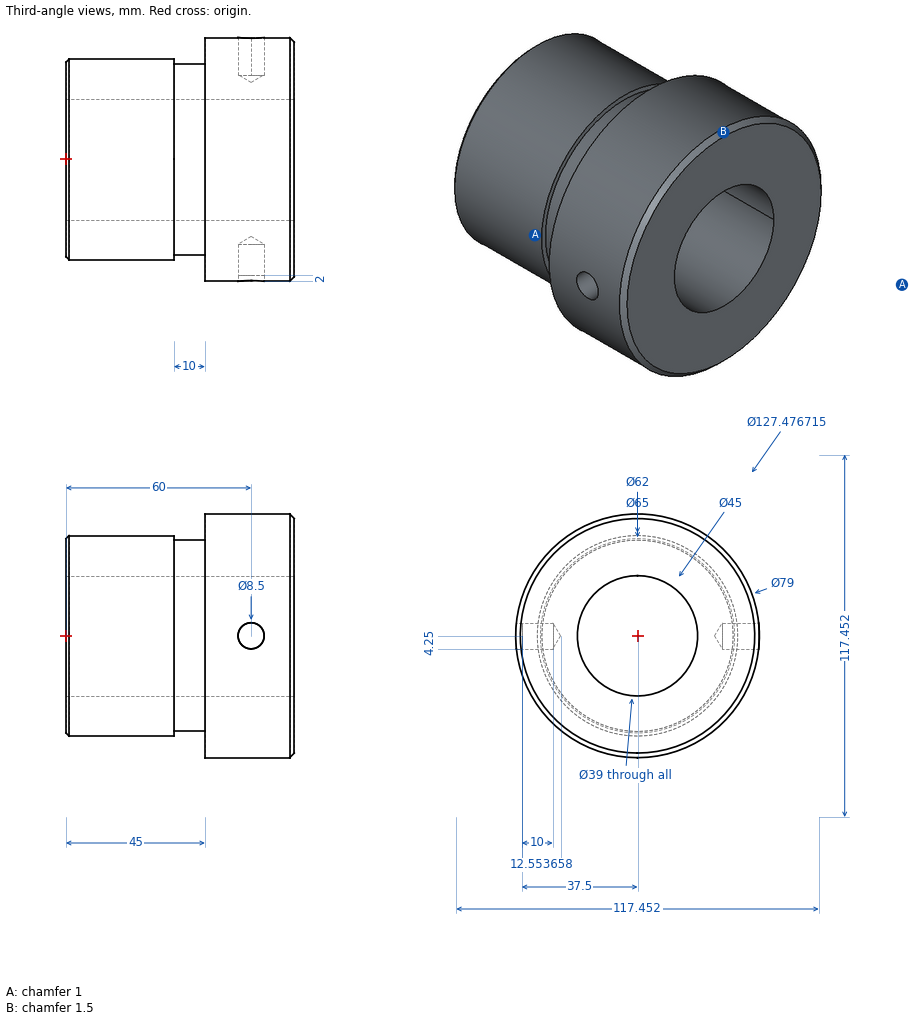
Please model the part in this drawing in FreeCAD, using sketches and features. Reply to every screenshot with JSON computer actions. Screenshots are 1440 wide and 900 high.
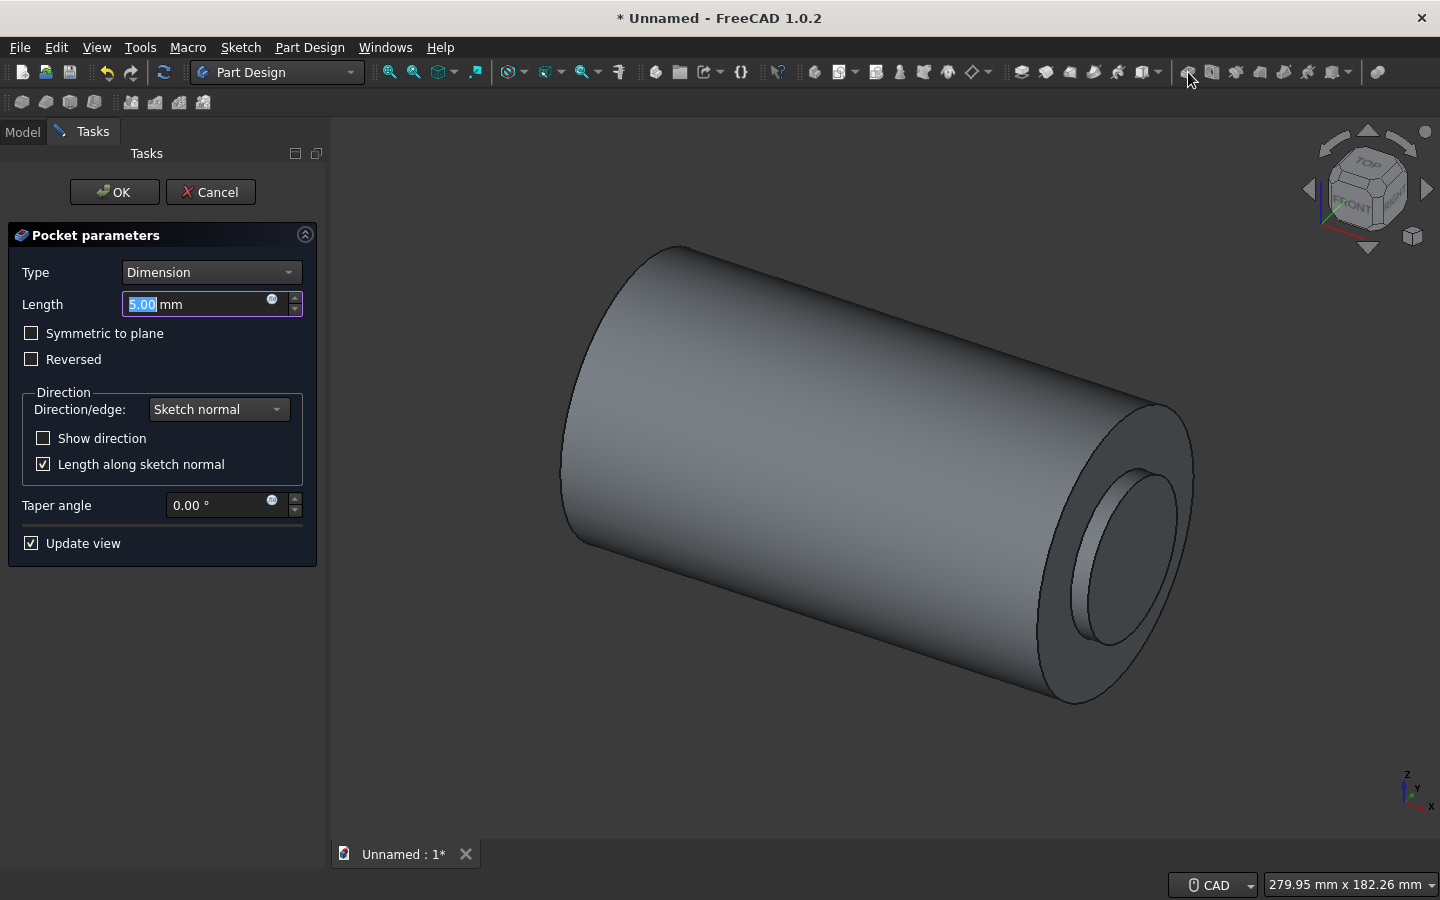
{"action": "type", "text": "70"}
{"action": "key", "text": "Tab"}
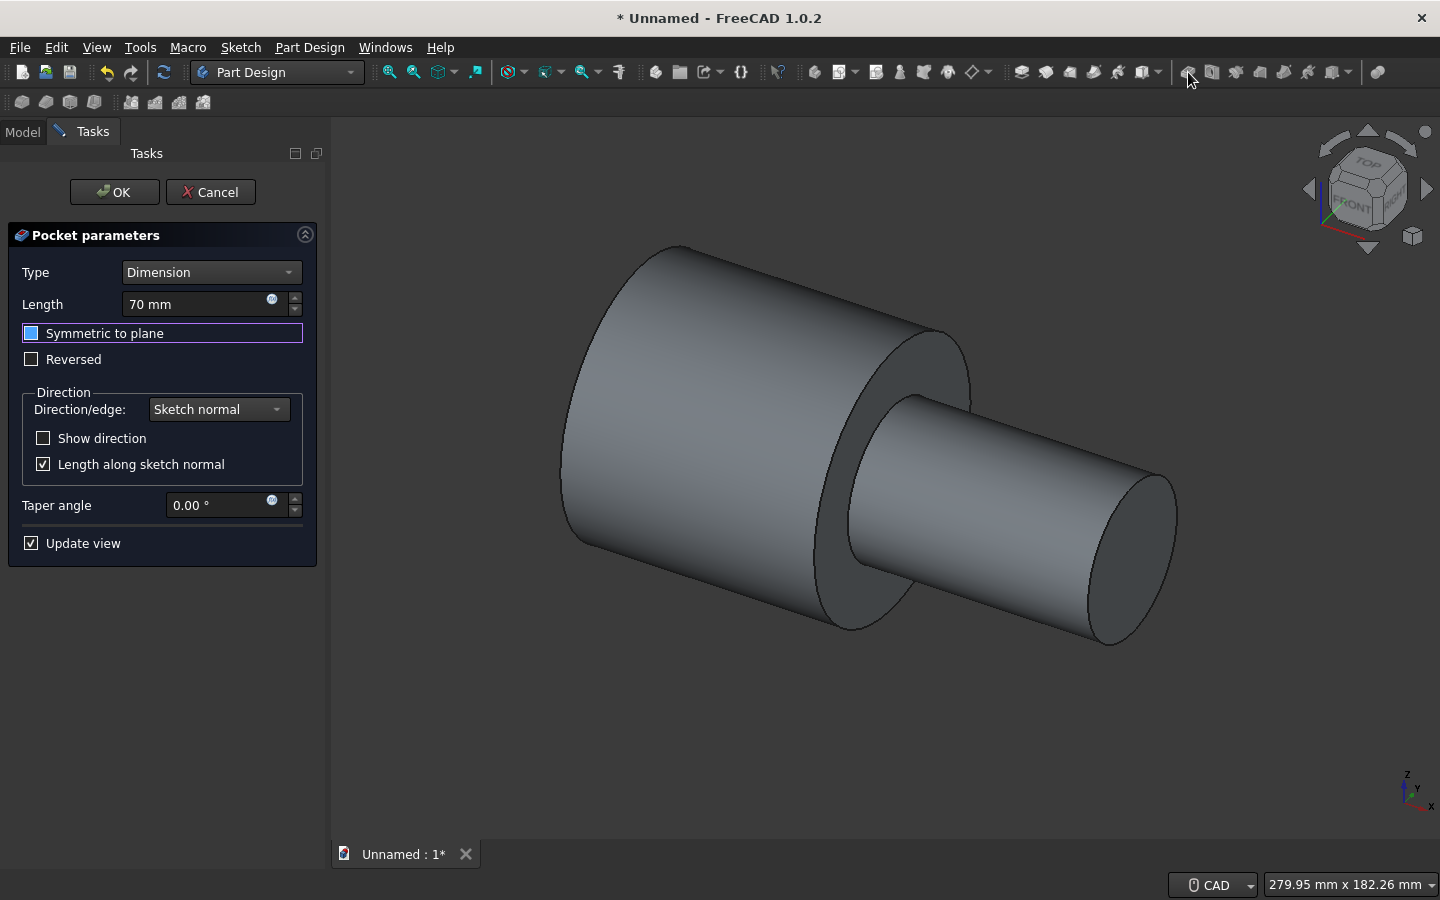
{"action": "left_click", "coordinate": [115, 192]}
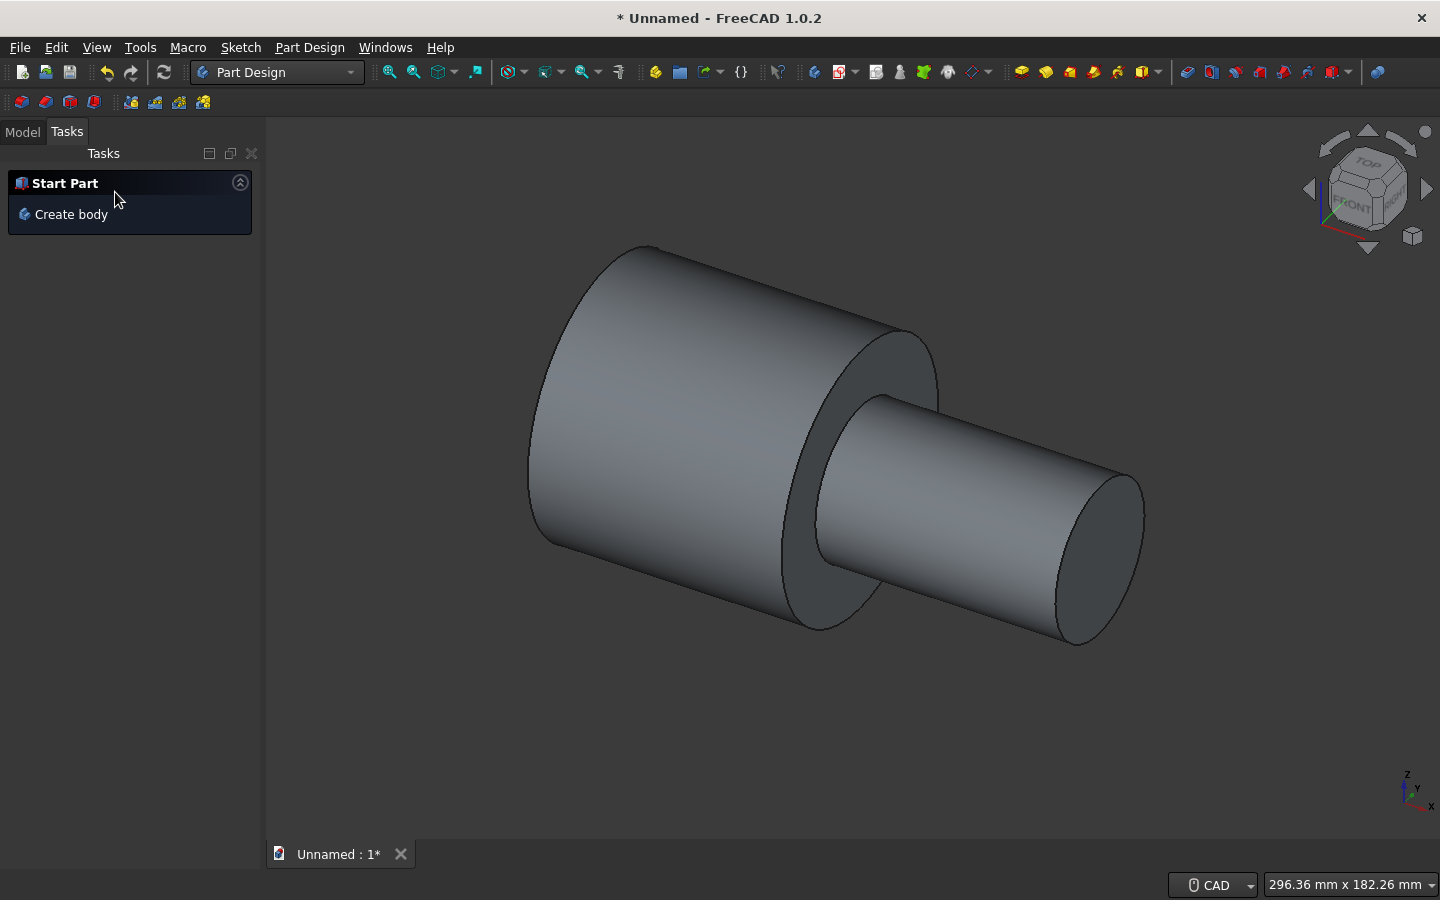
{"action": "key", "text": "6"}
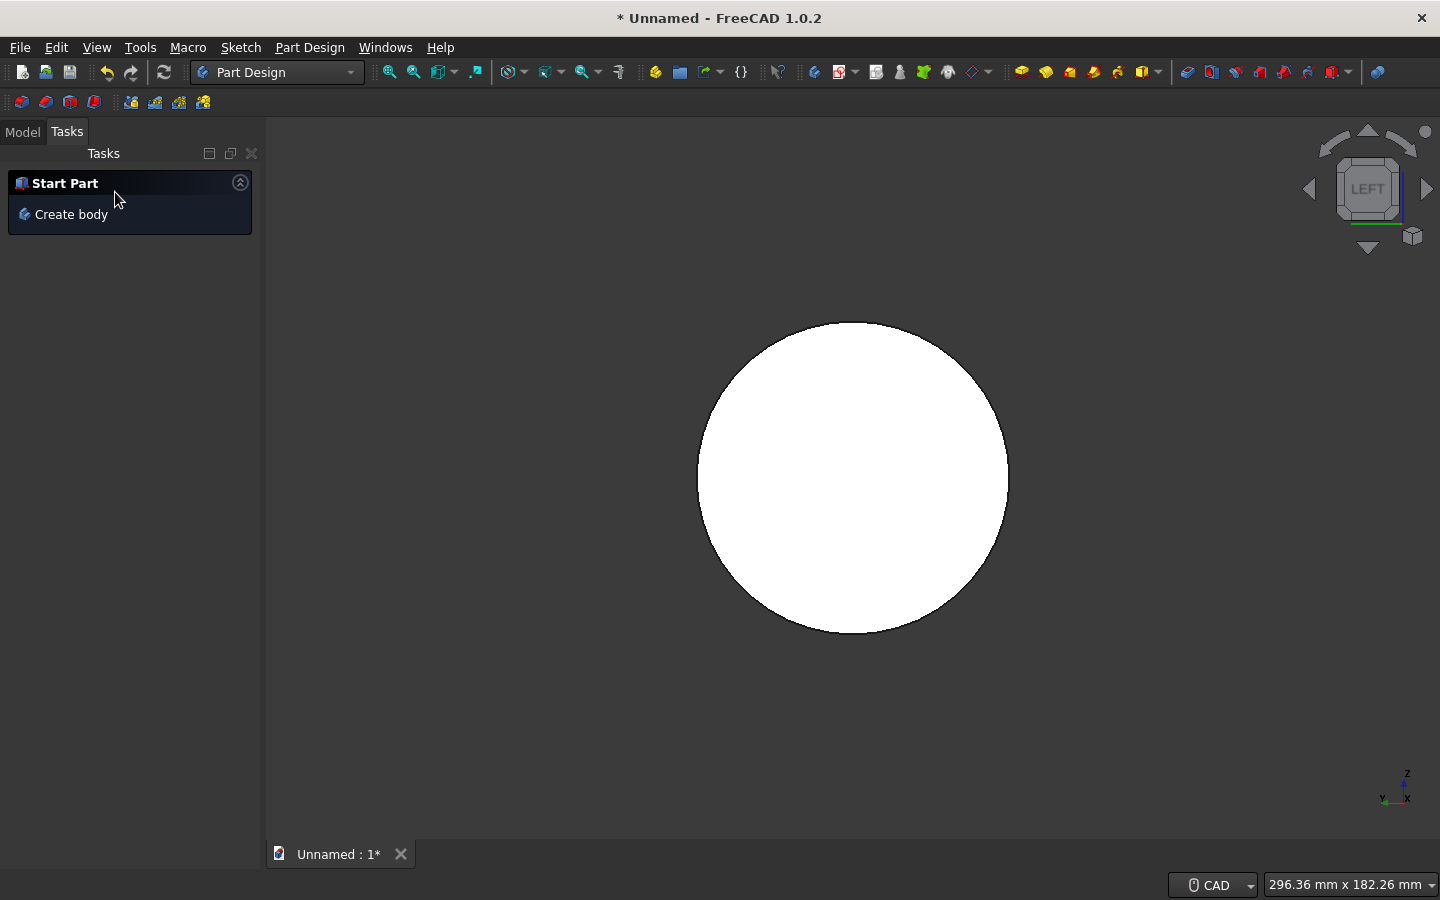
{"action": "key", "text": "v f"}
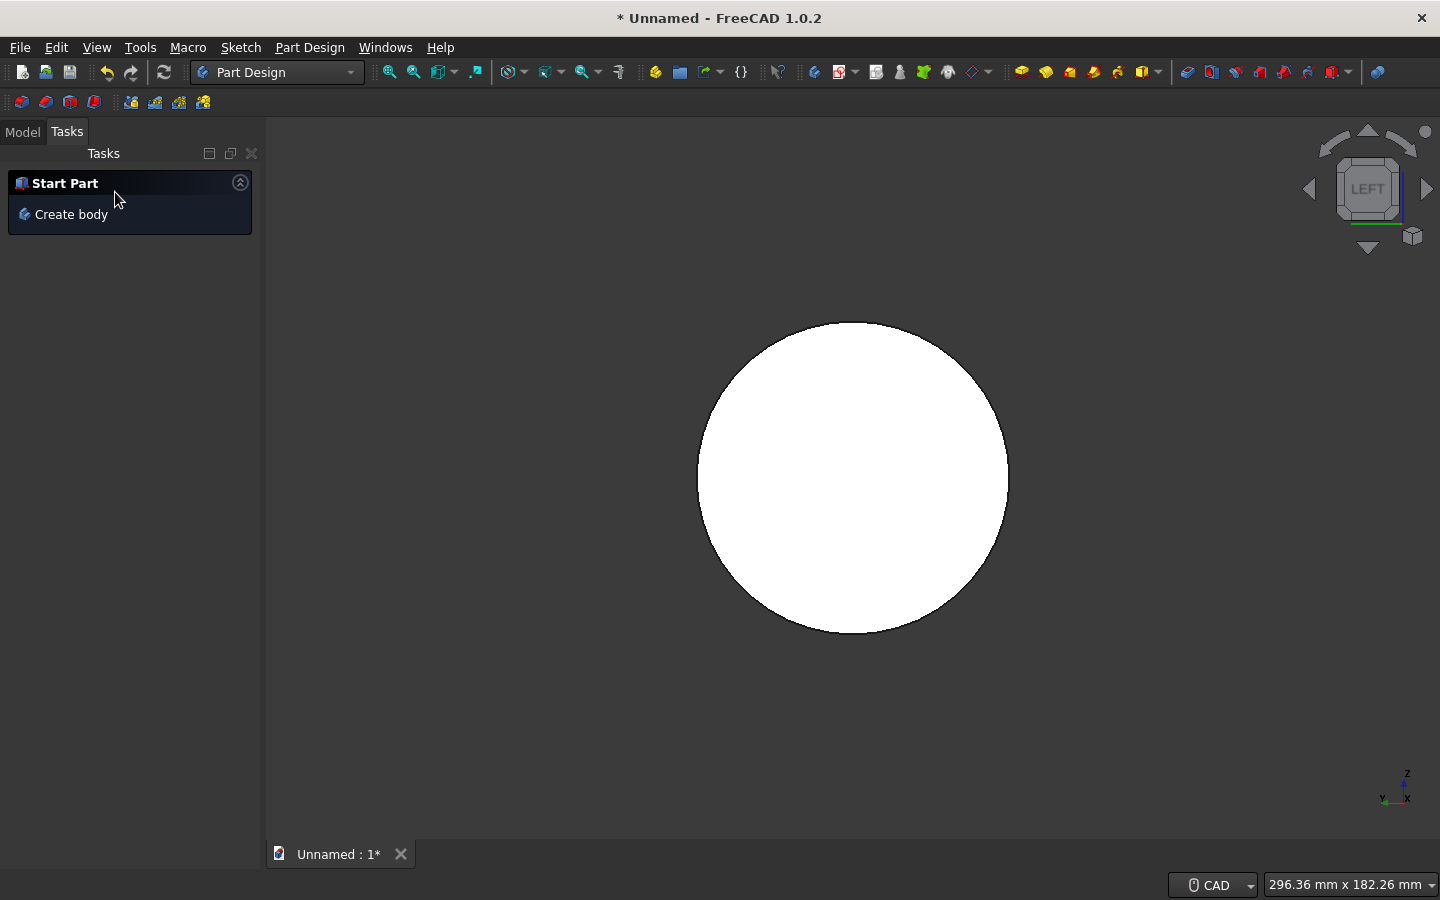
{"action": "left_click", "coordinate": [853, 477]}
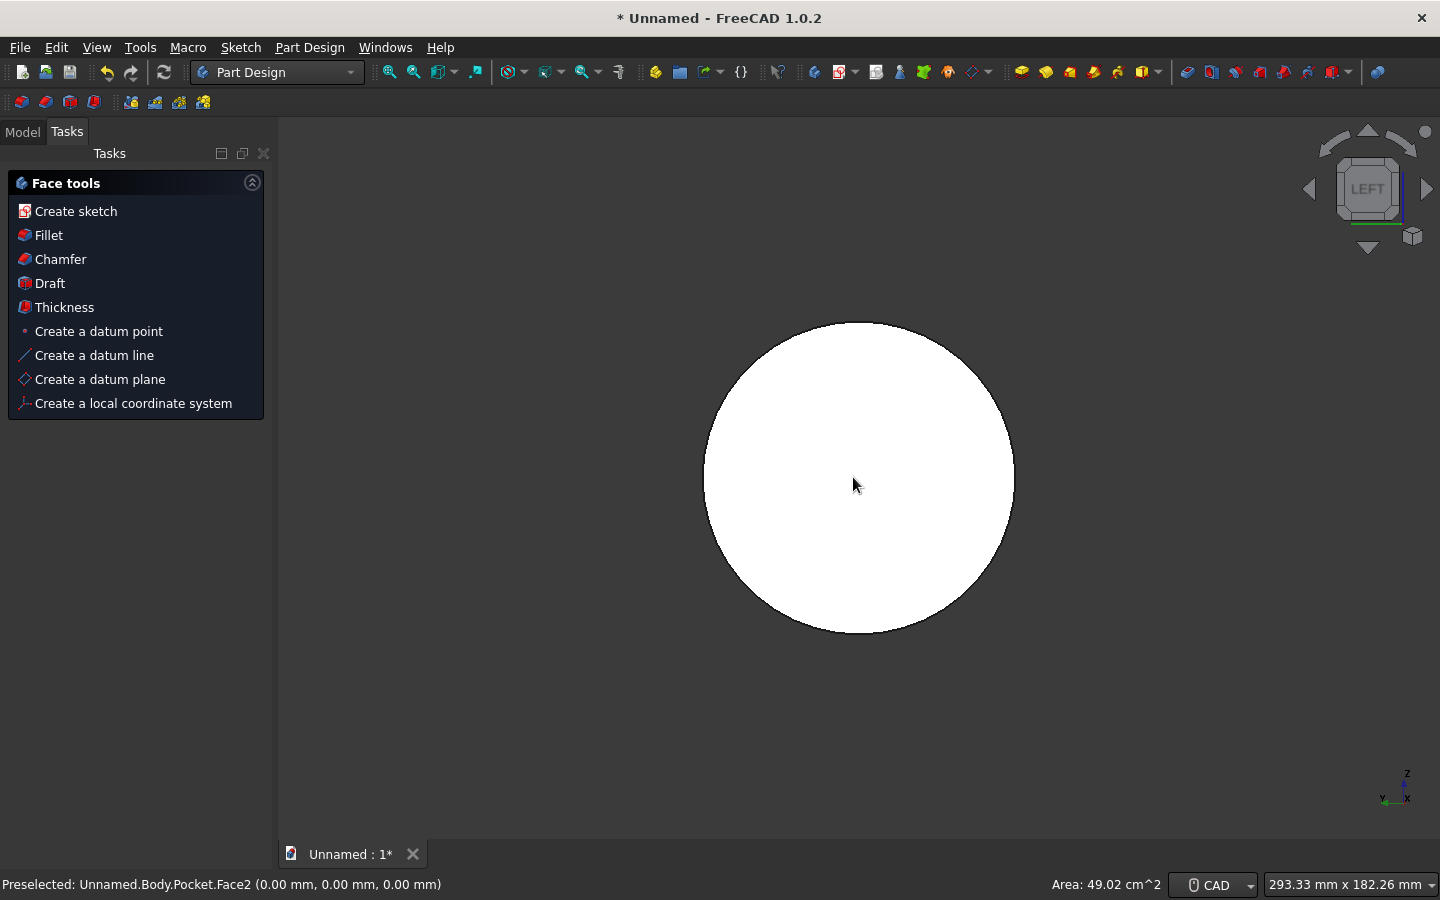
{"action": "left_click", "coordinate": [840, 72]}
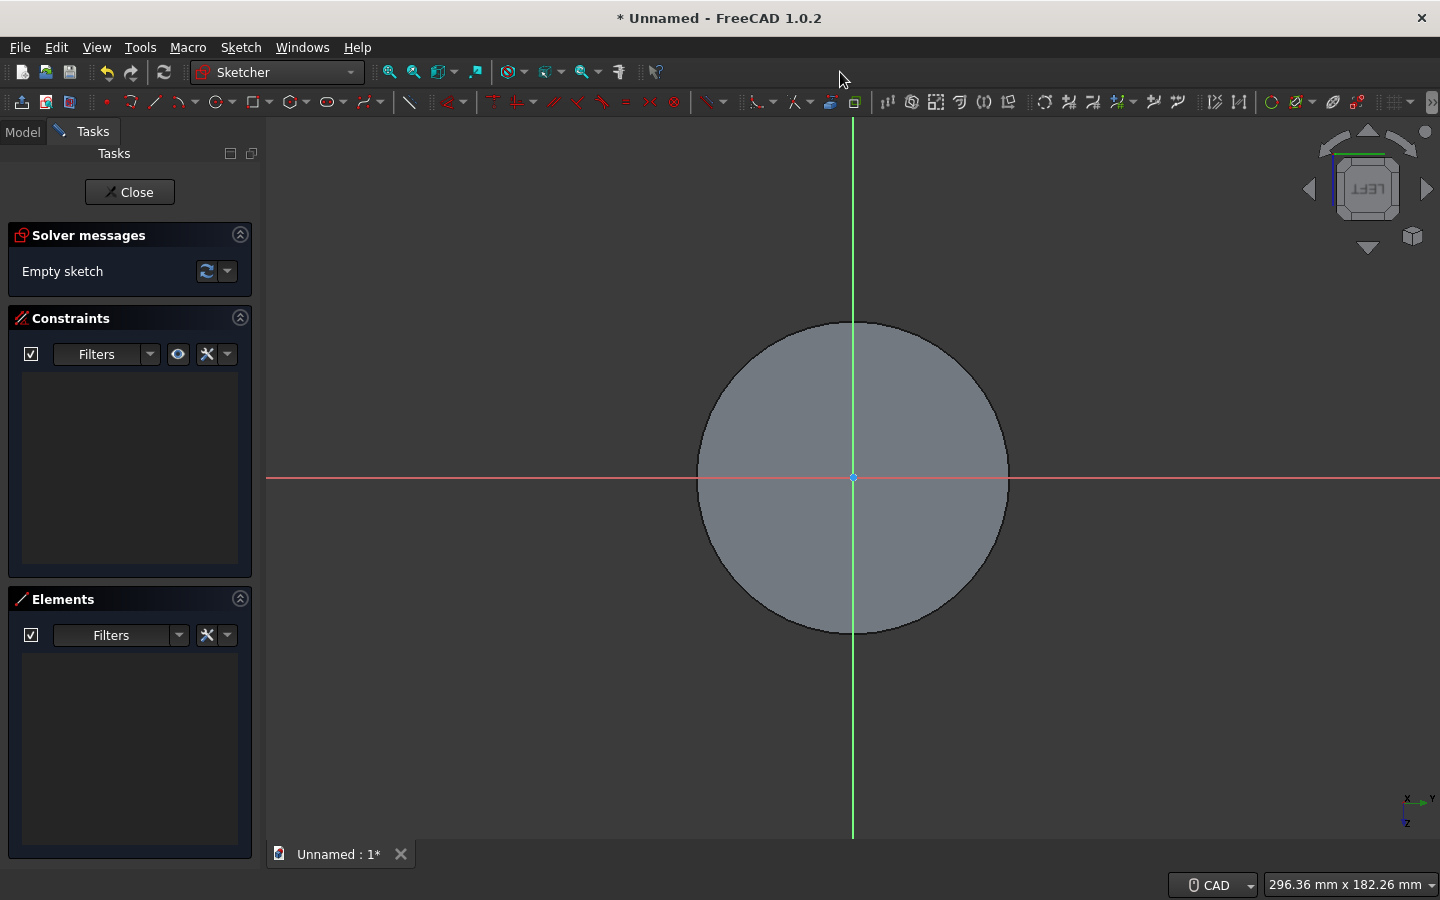
{"action": "key", "text": "g v"}